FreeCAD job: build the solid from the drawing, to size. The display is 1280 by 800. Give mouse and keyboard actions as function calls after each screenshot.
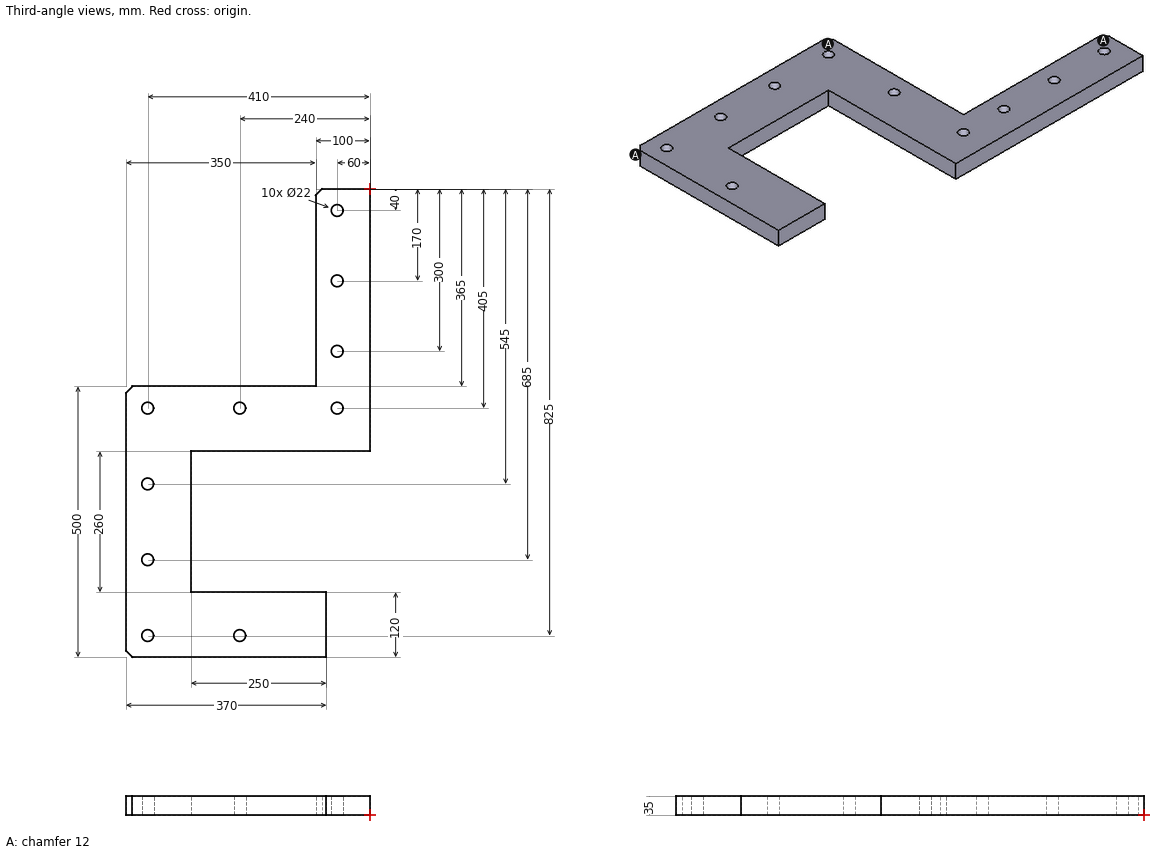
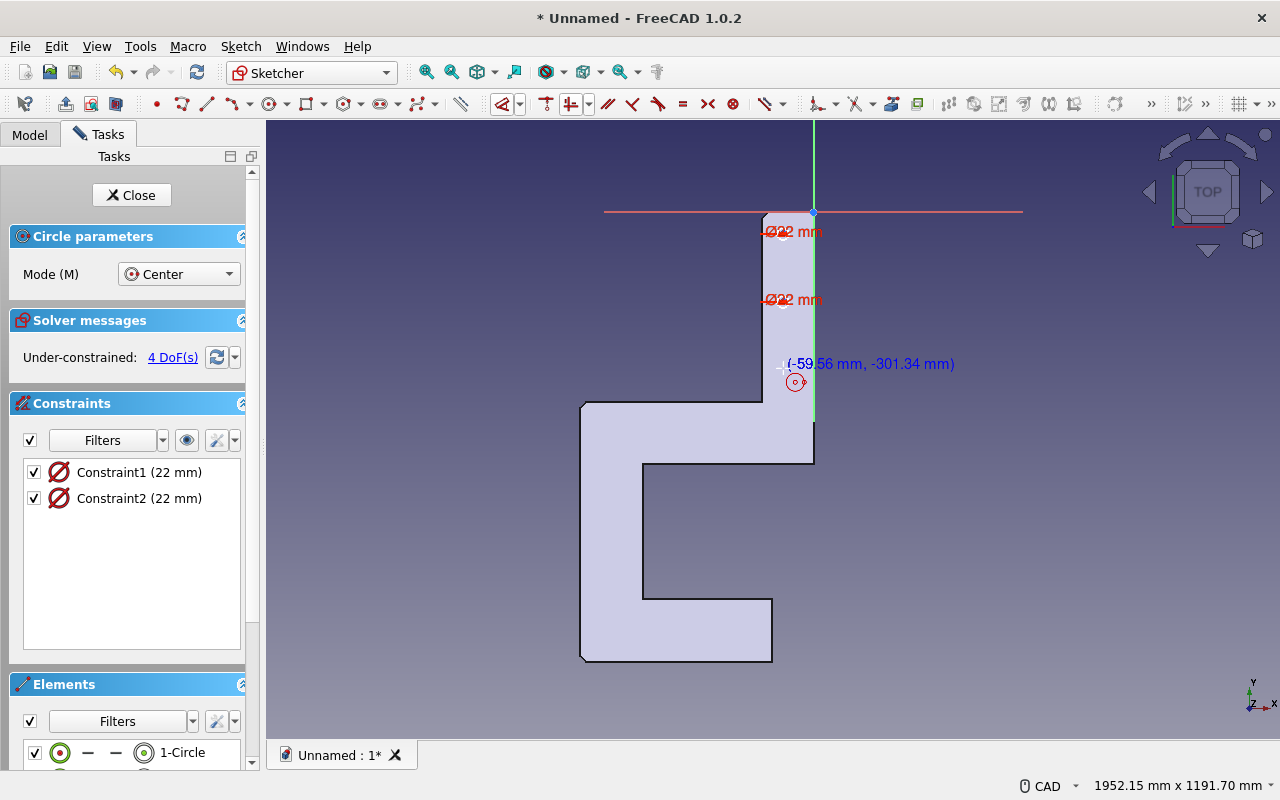
click(783, 368)
move(787, 364)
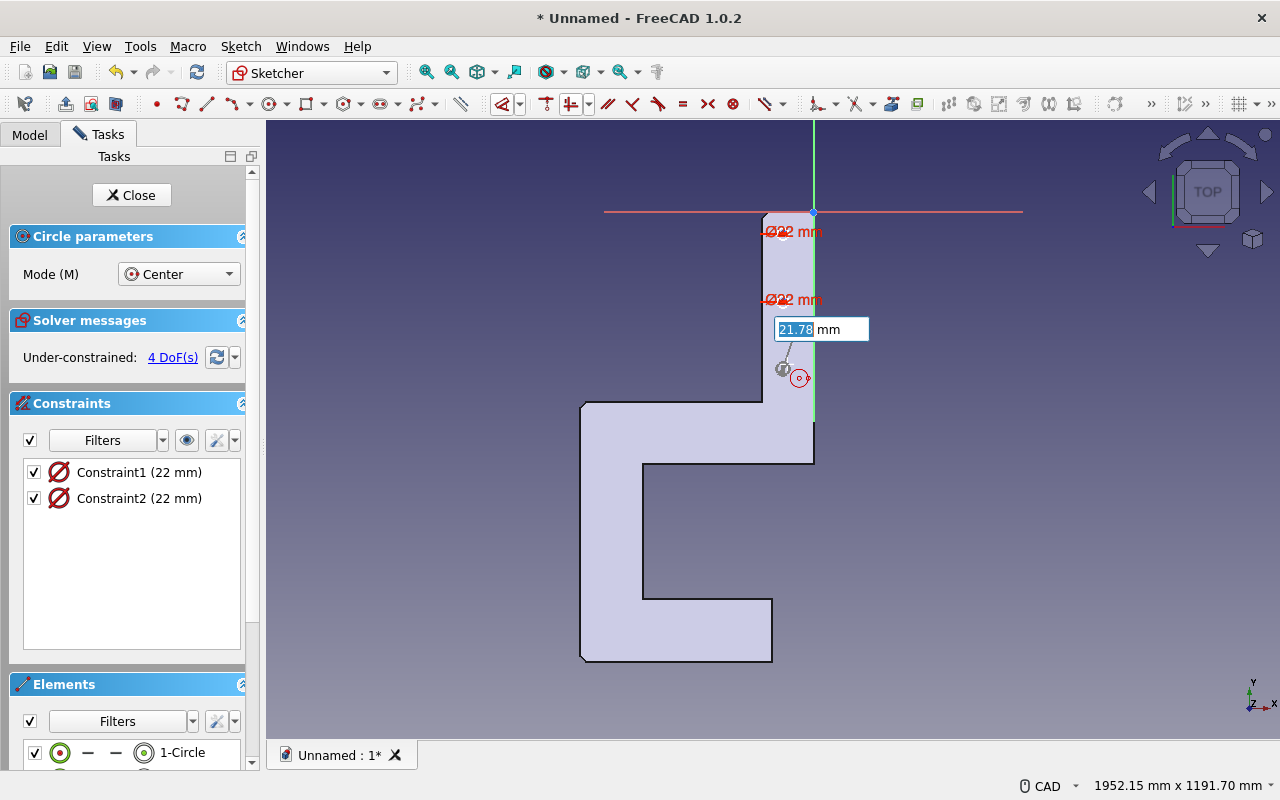
text(22)
key(Return)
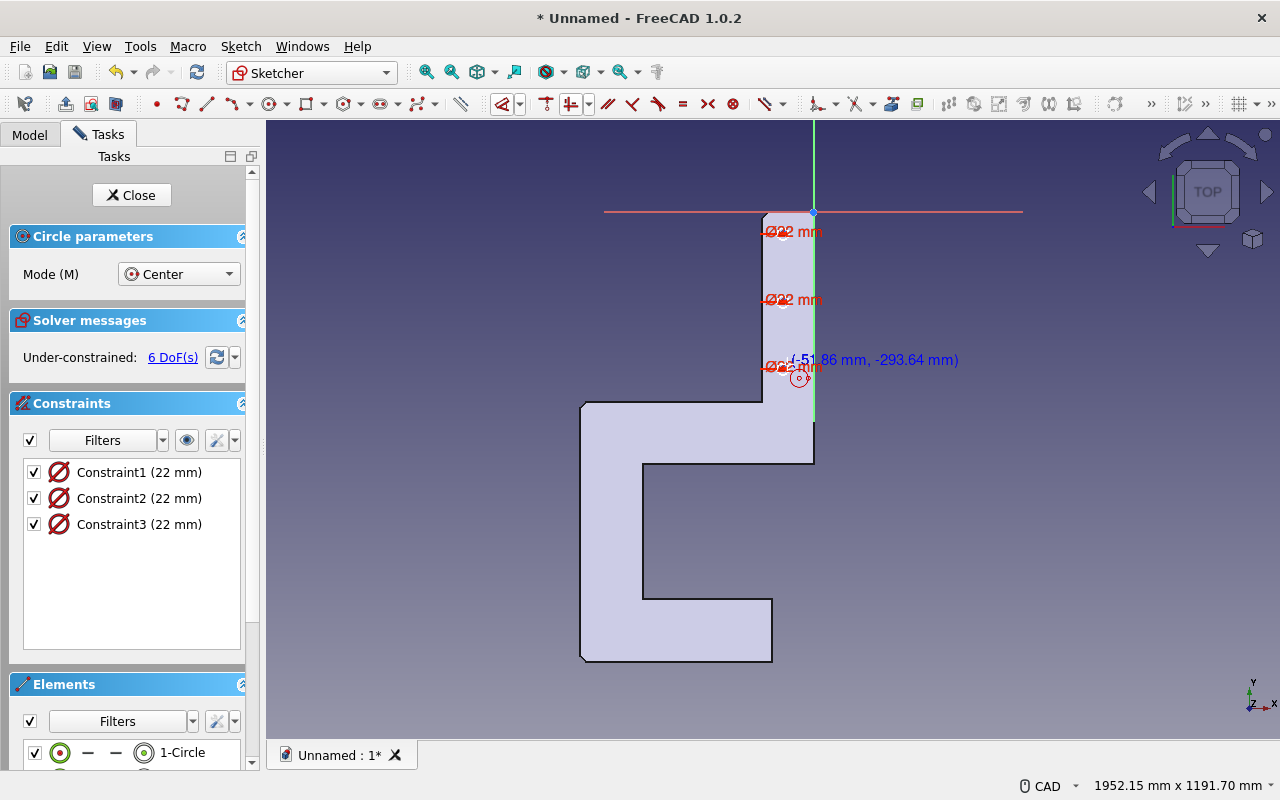
scroll(783, 423, up, 7)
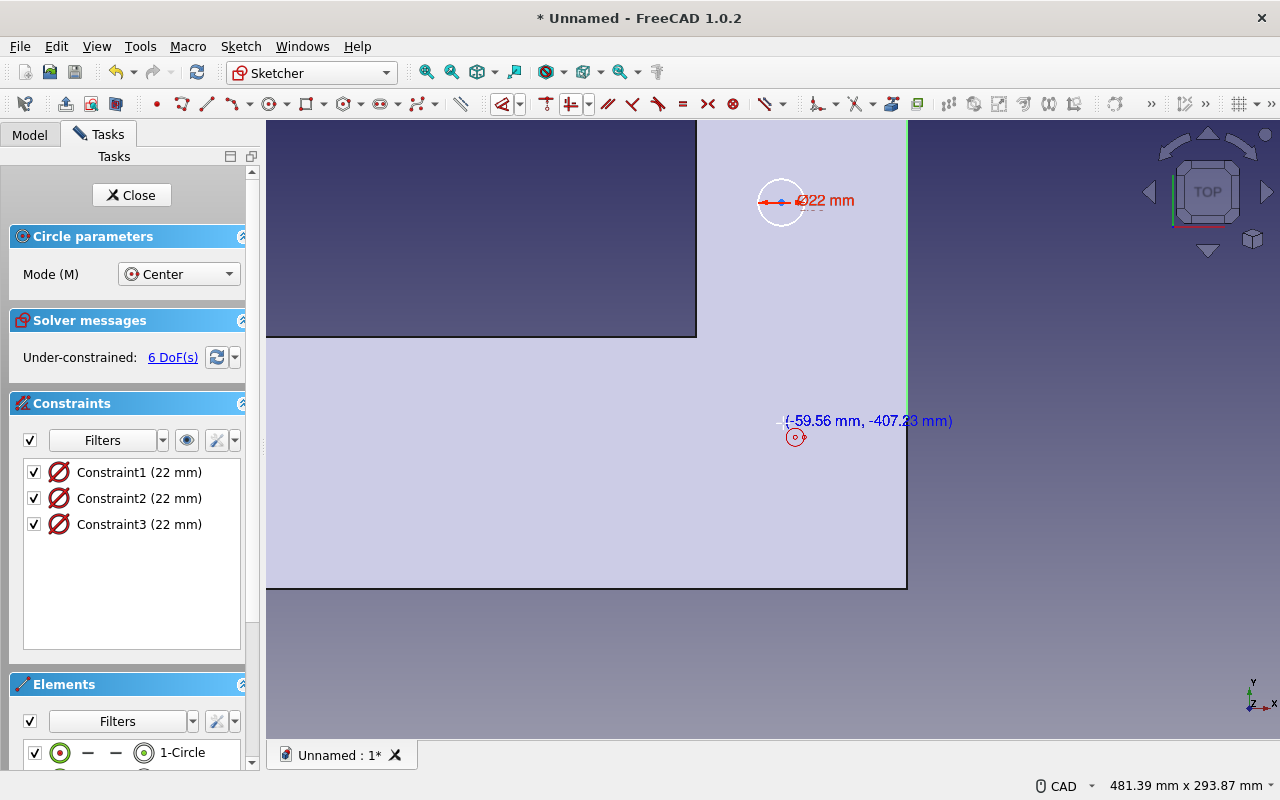
scroll(783, 423, down, 7)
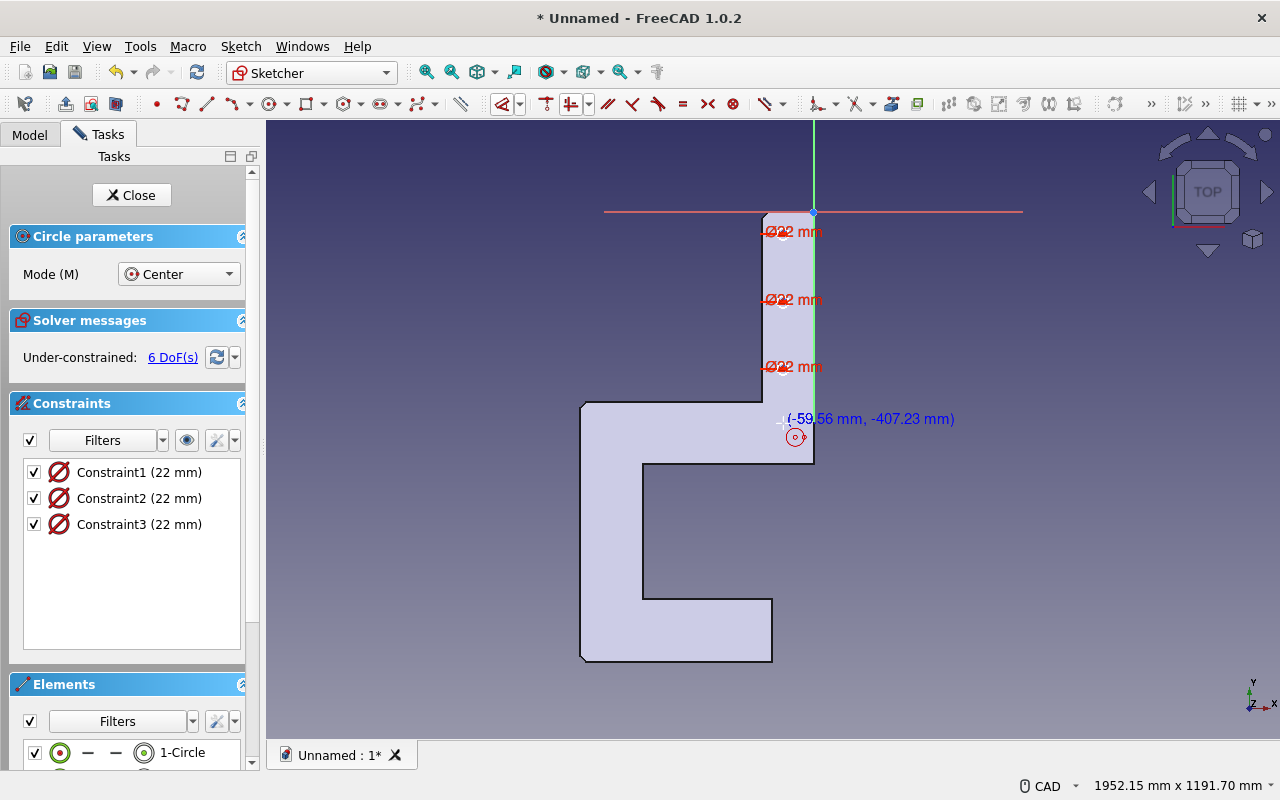
click(783, 423)
move(787, 419)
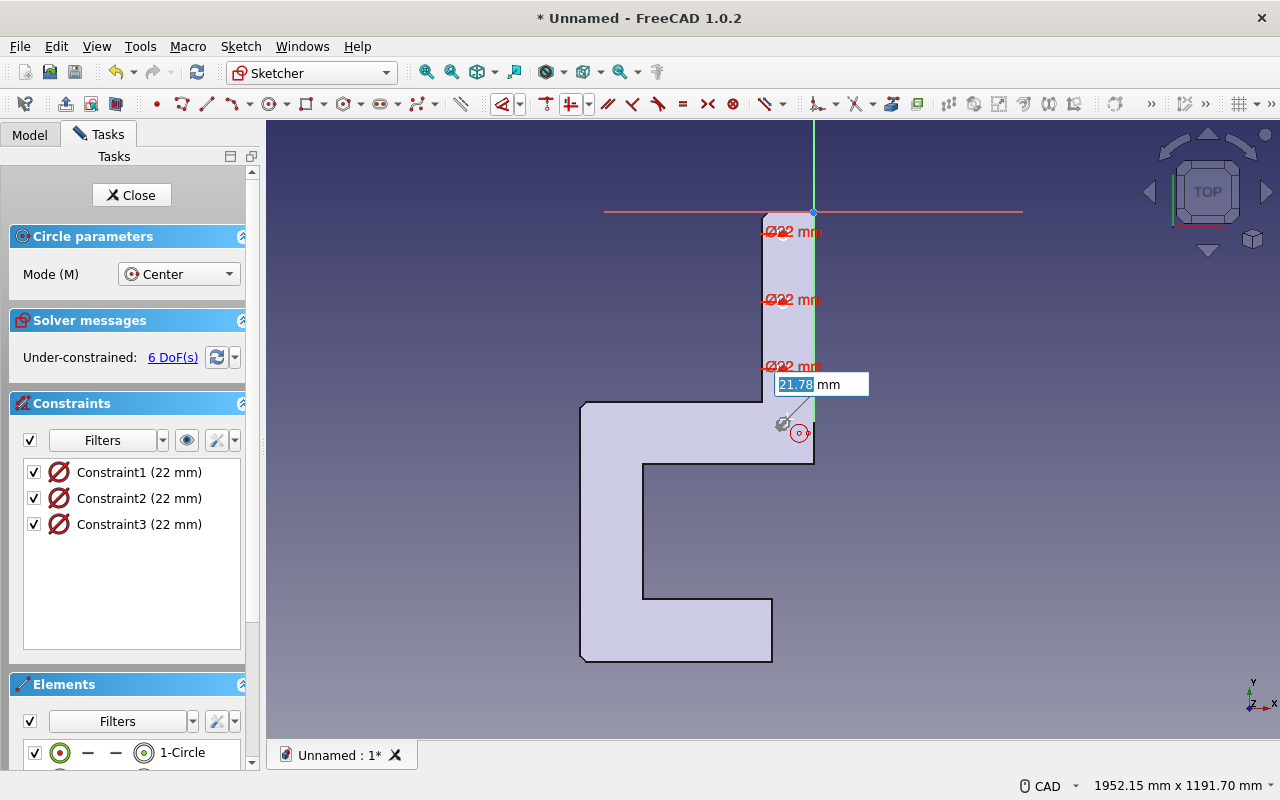
text(22)
key(Return)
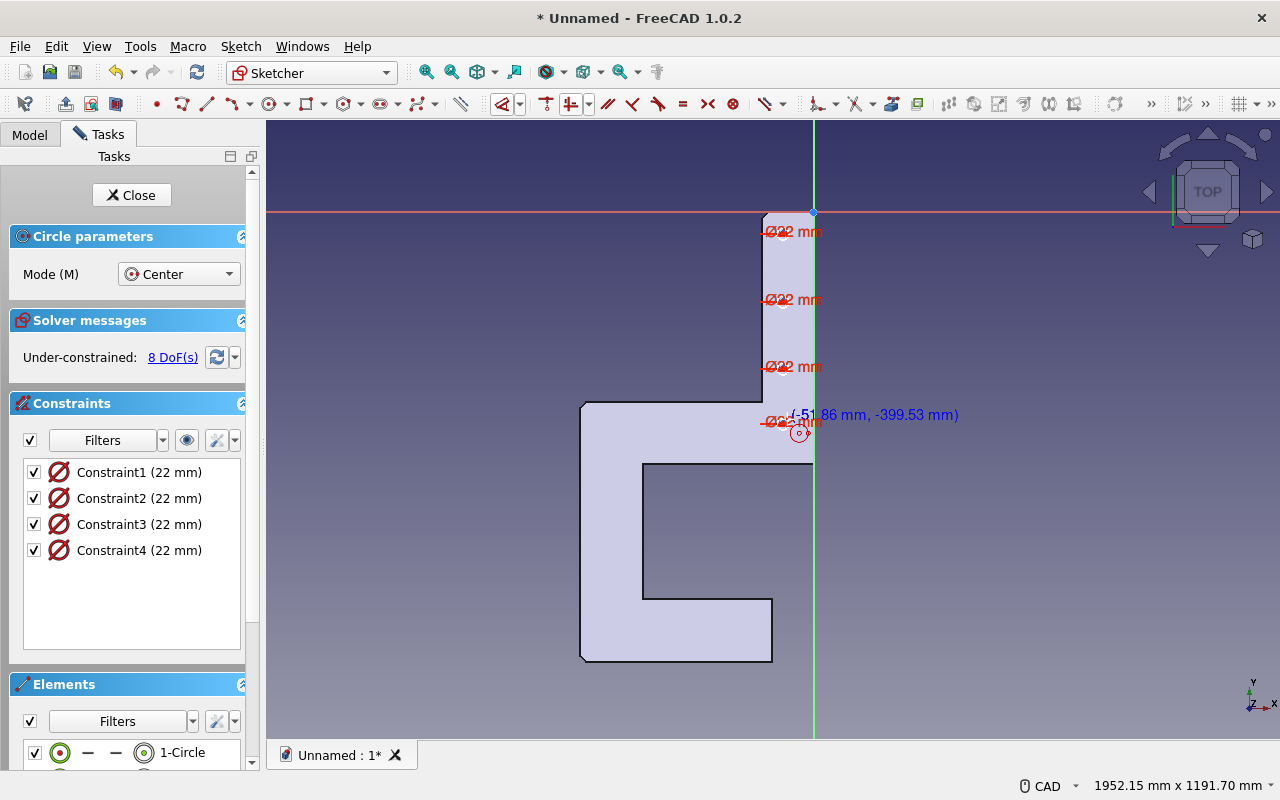
scroll(689, 423, up, 7)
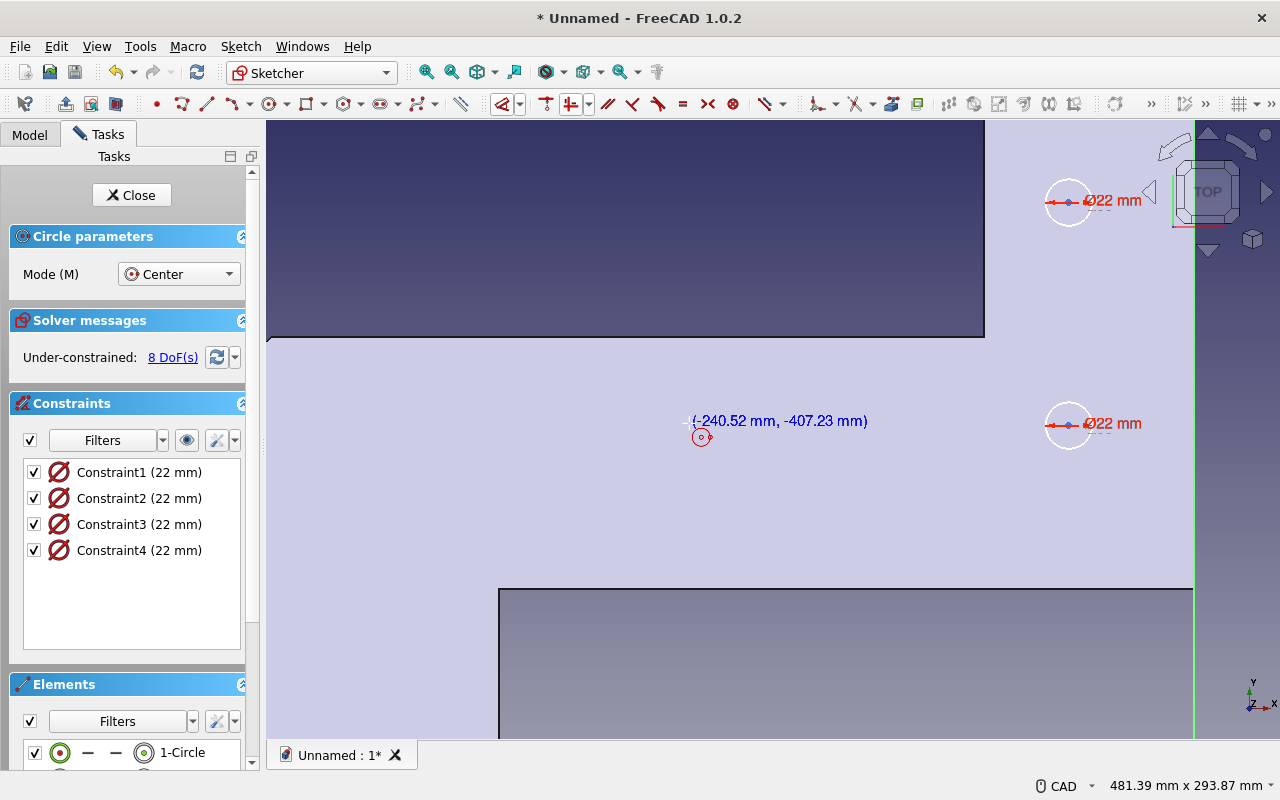
scroll(689, 423, down, 7)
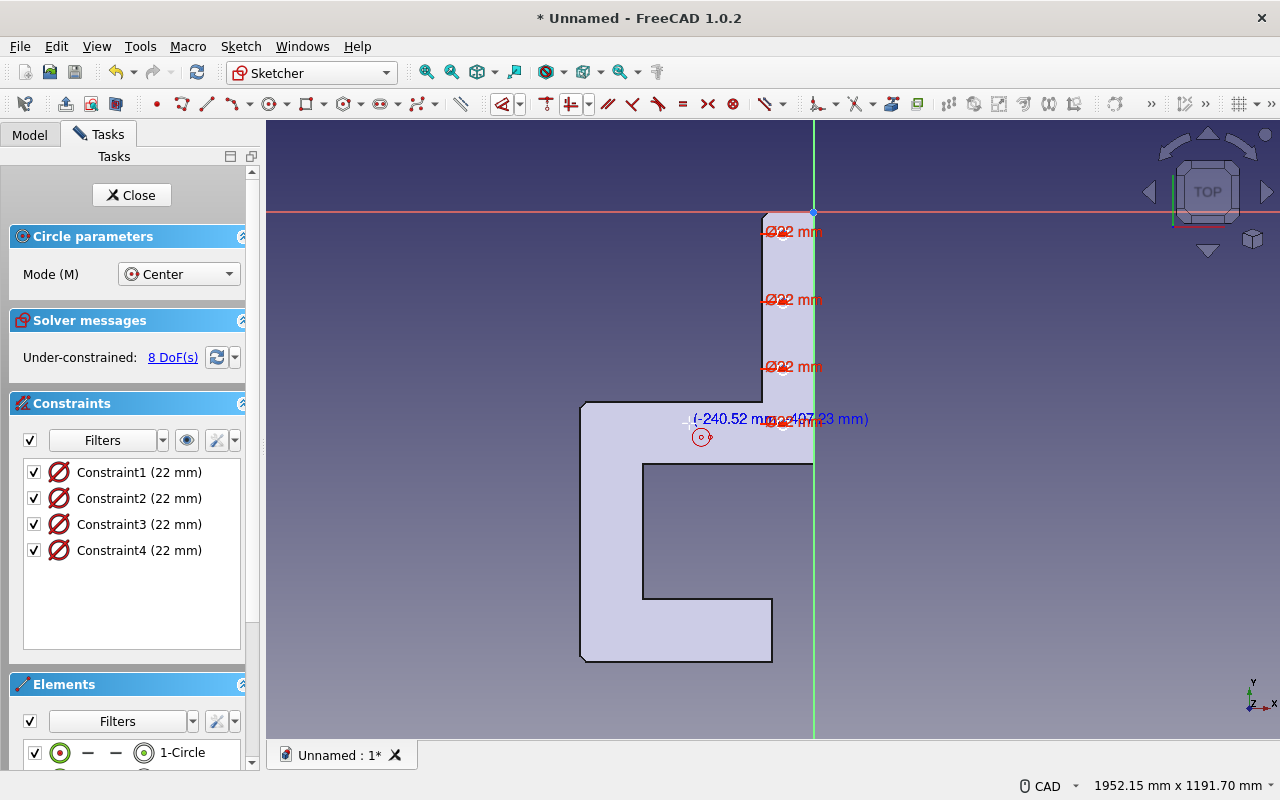
click(689, 423)
move(693, 419)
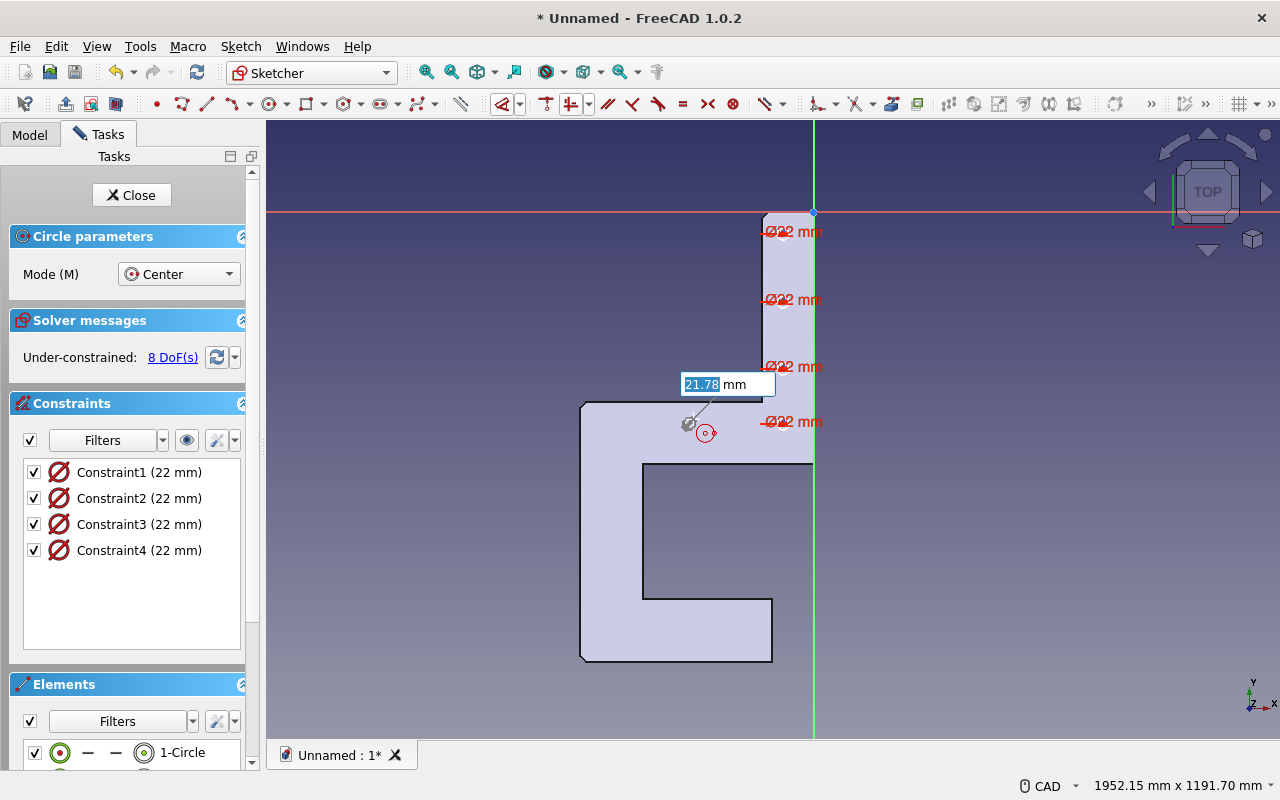
text(22)
key(Return)